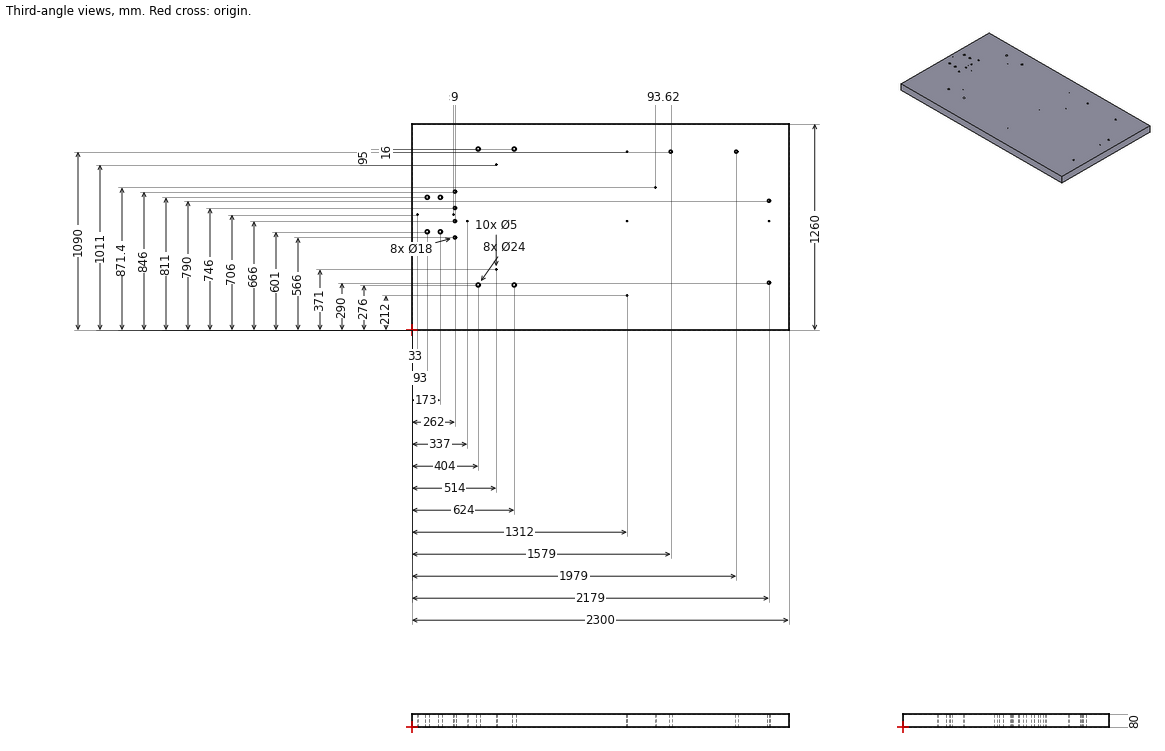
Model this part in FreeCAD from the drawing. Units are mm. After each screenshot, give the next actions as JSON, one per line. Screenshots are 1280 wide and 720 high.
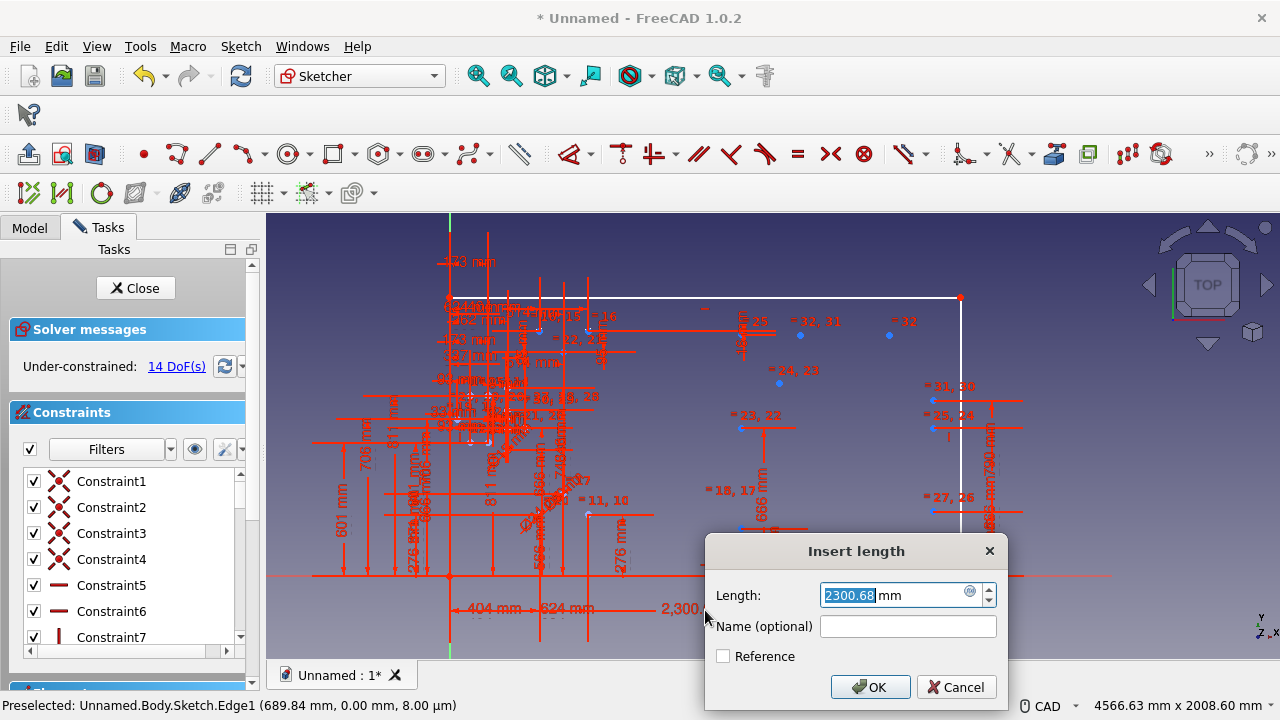
{"action": "type", "text": "2300"}
{"action": "key", "text": "Return"}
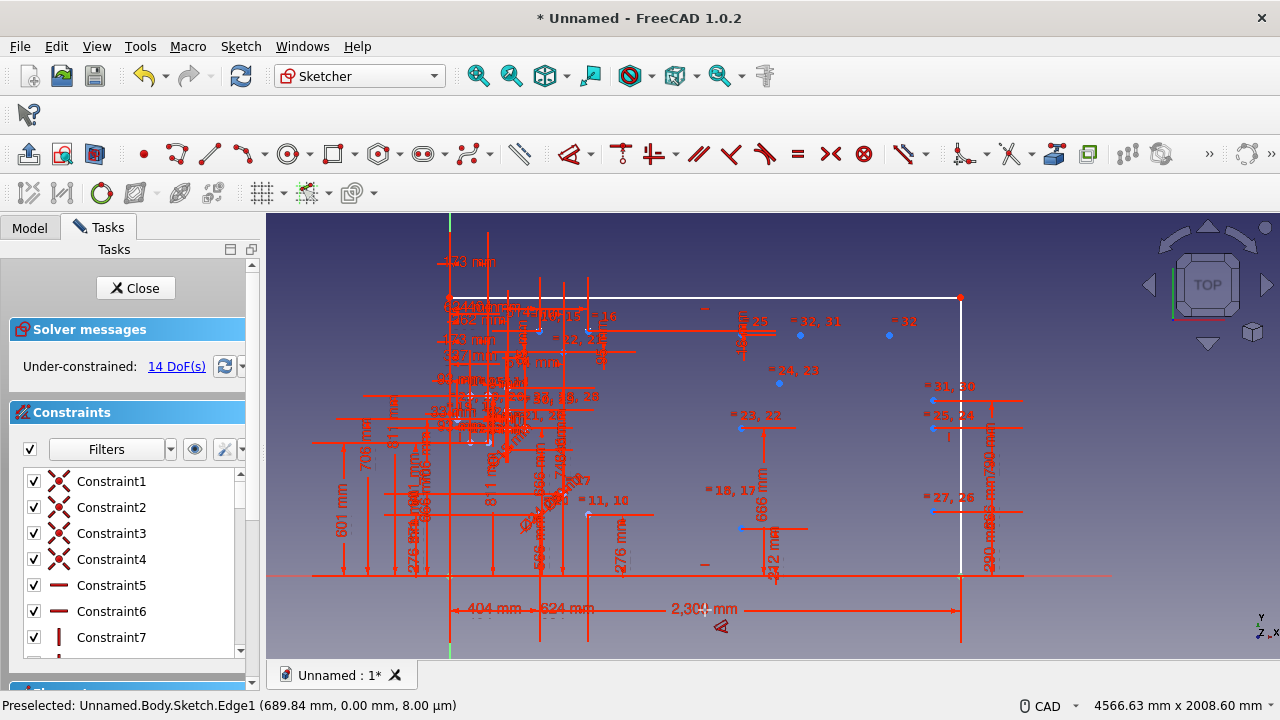
{"action": "left_click", "coordinate": [961, 493]}
{"action": "left_click", "coordinate": [995, 373]}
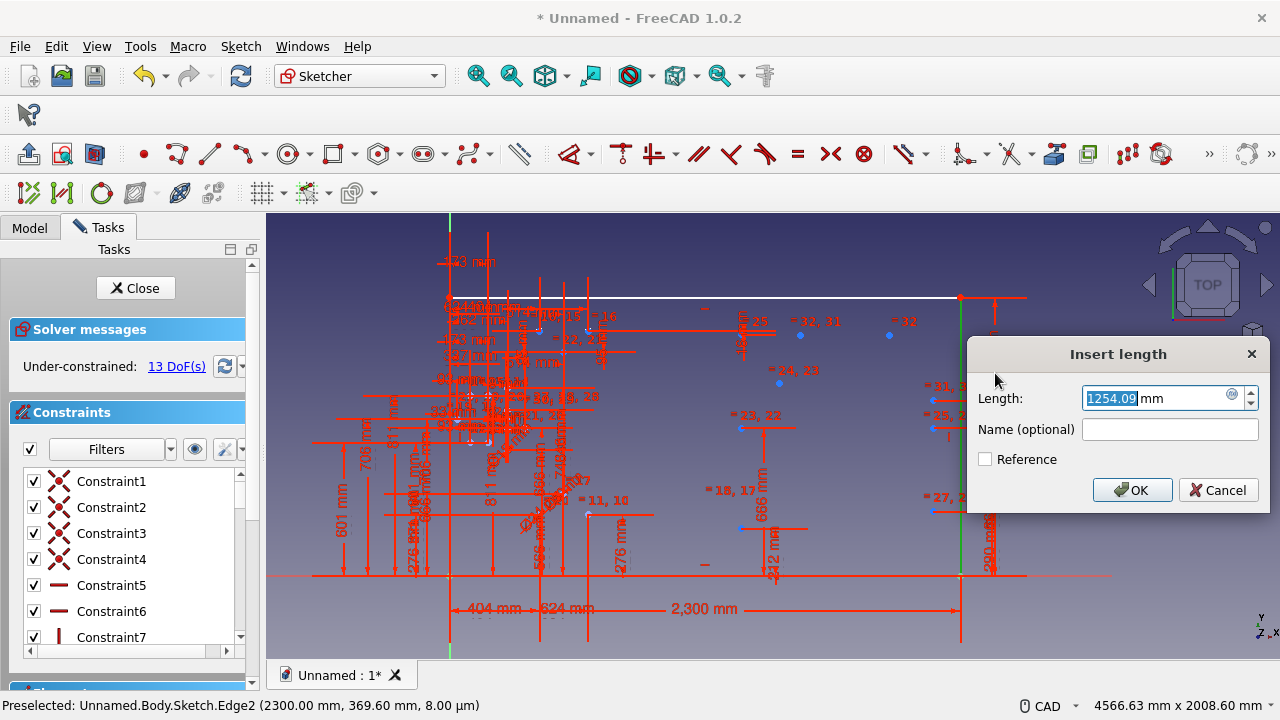
{"action": "type", "text": "1260"}
{"action": "key", "text": "Return"}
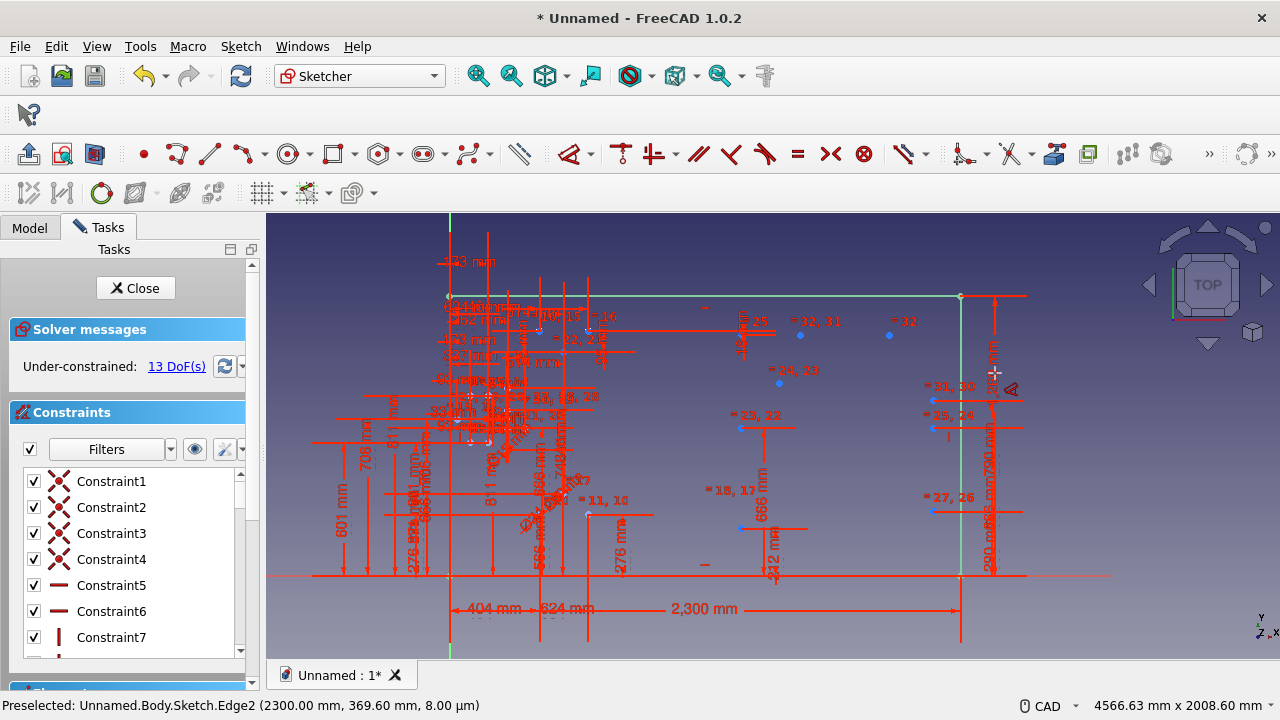
{"action": "left_click", "coordinate": [741, 529]}
{"action": "left_click", "coordinate": [663, 495]}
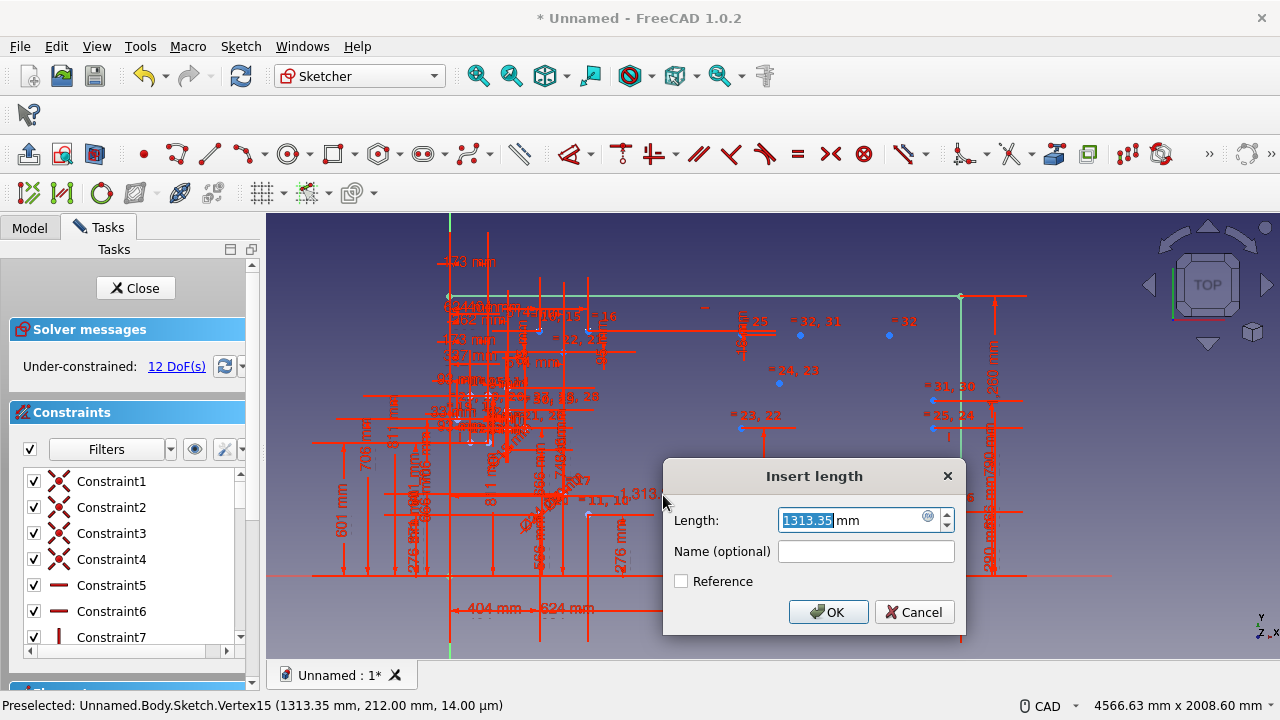
{"action": "type", "text": "1312"}
{"action": "key", "text": "Return"}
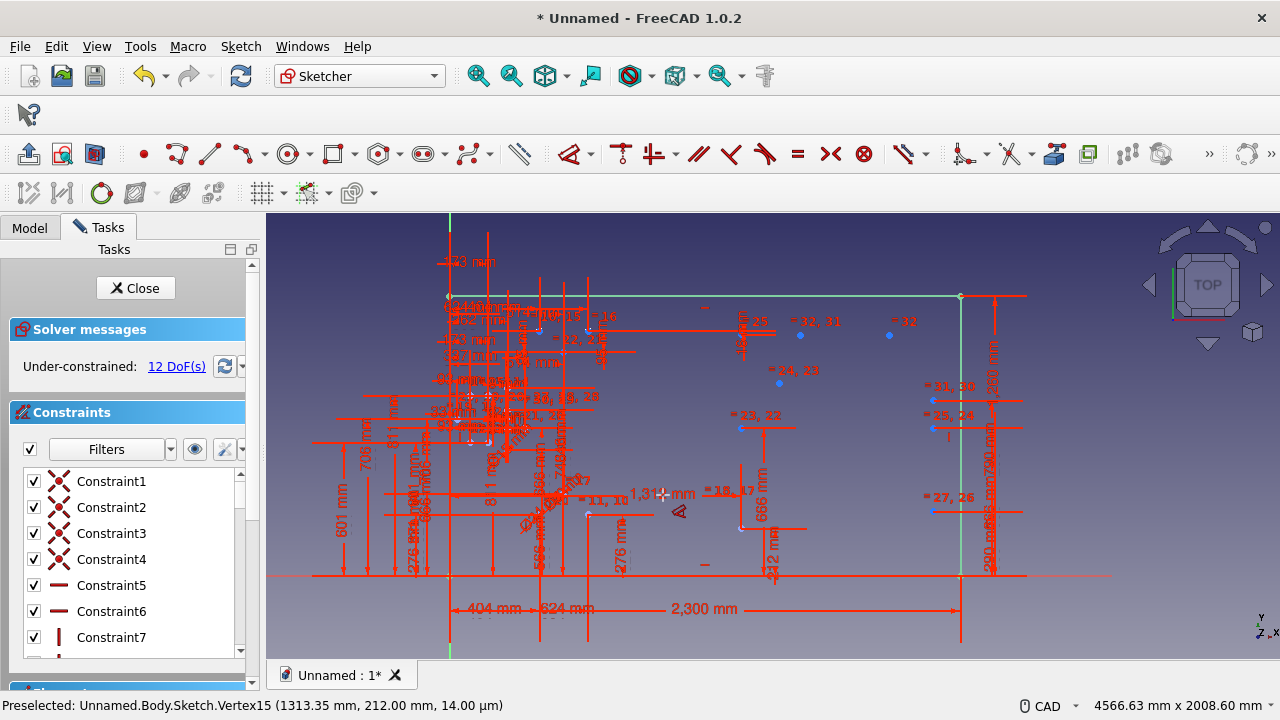
{"action": "left_click", "coordinate": [933, 512]}
{"action": "left_click", "coordinate": [803, 610]}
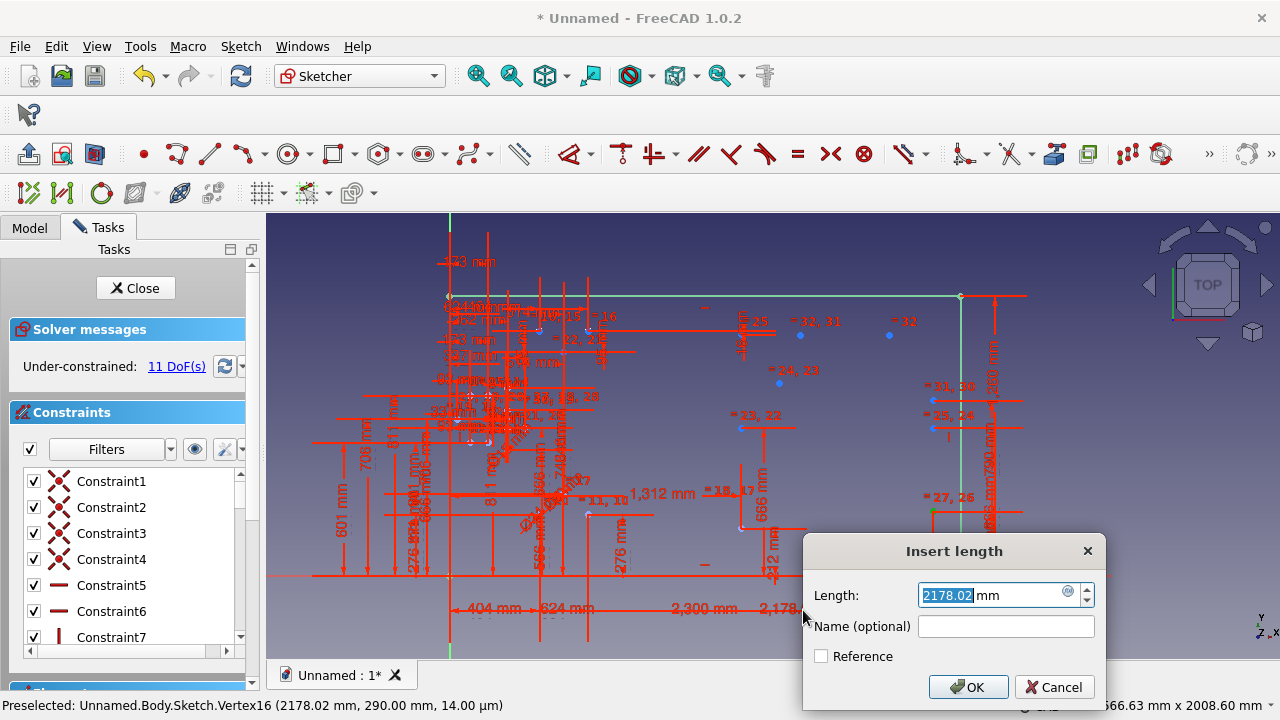
{"action": "type", "text": "2179"}
{"action": "key", "text": "Return"}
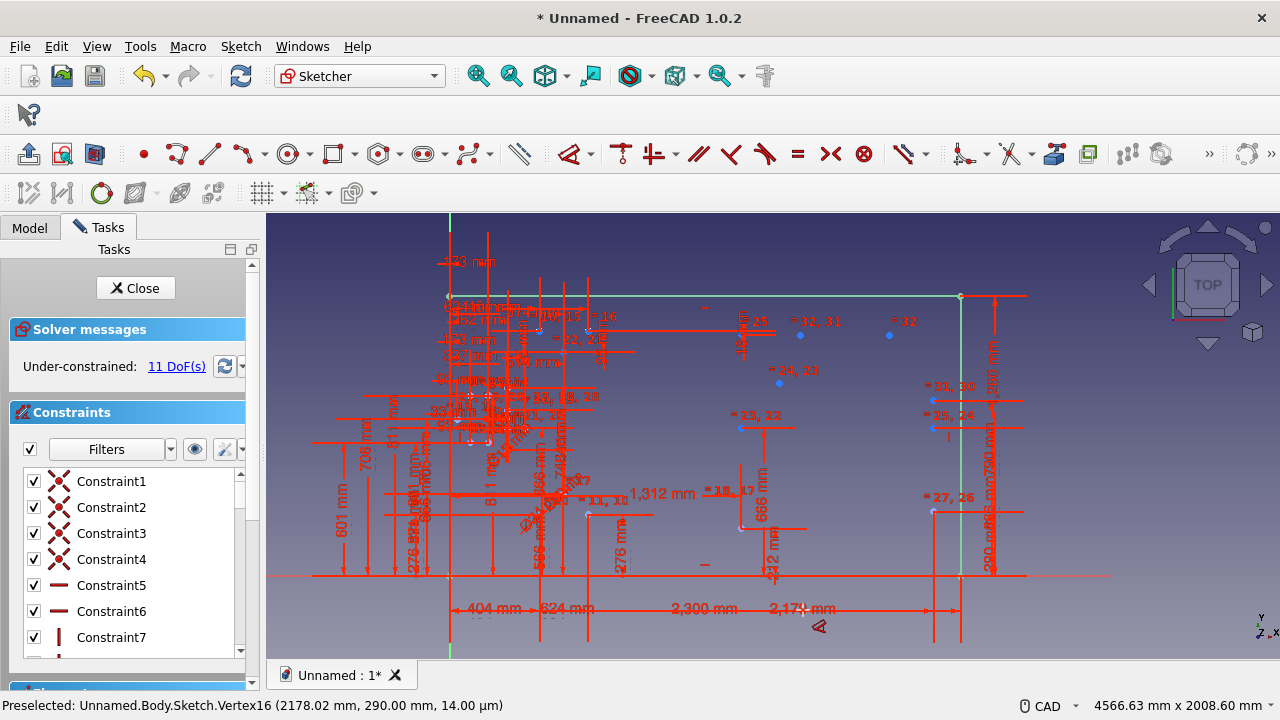
{"action": "left_click", "coordinate": [564, 352]}
{"action": "left_click", "coordinate": [598, 413]}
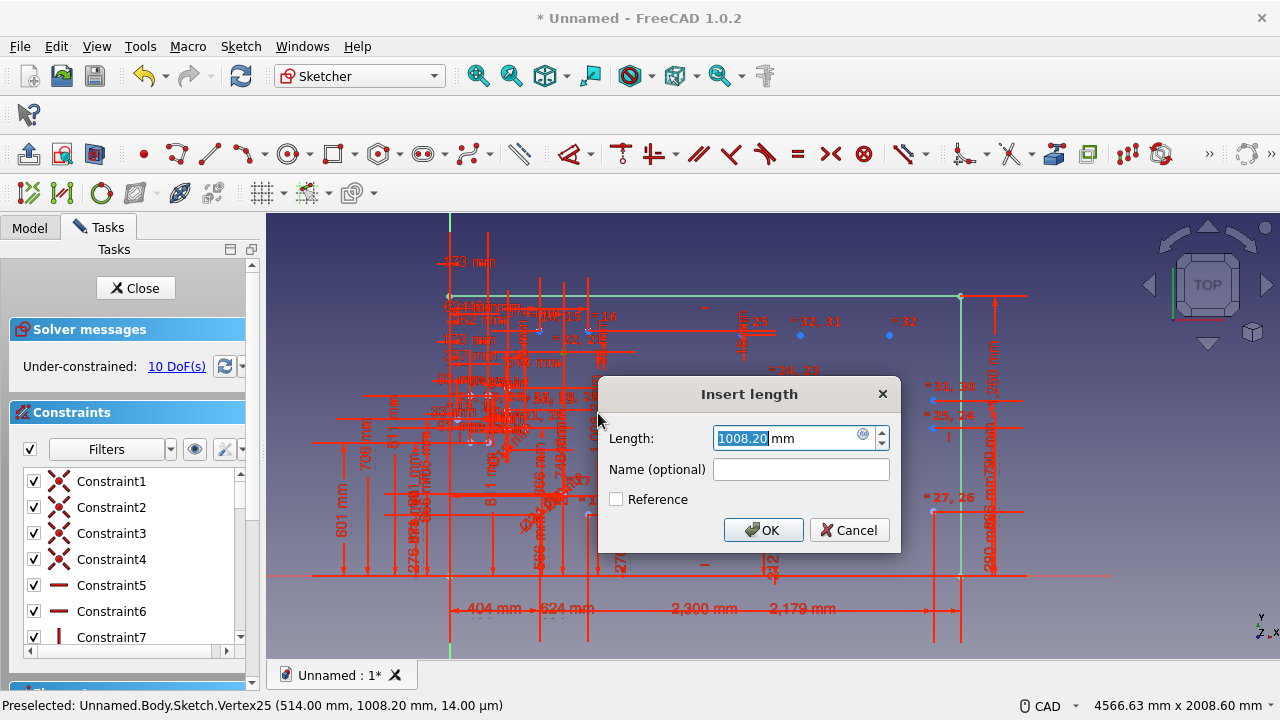
{"action": "type", "text": "1011"}
{"action": "key", "text": "Return"}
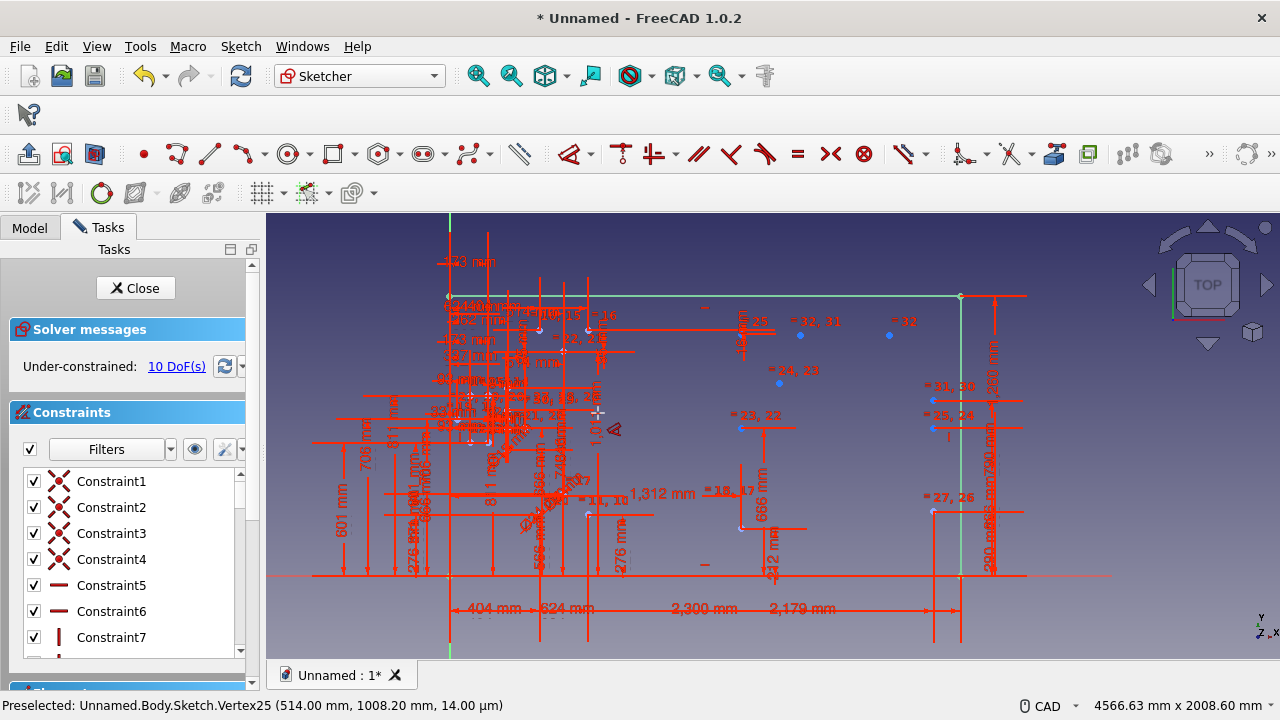
{"action": "left_click", "coordinate": [741, 428]}
{"action": "left_click", "coordinate": [697, 394]}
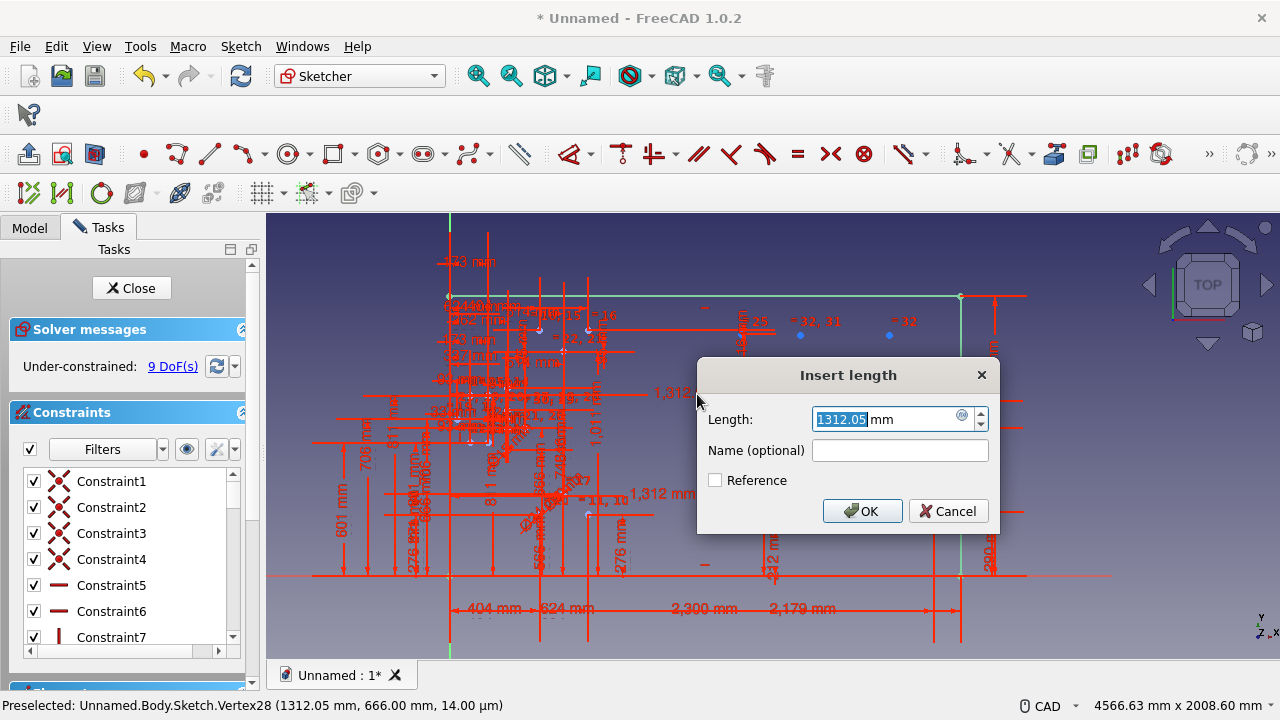
{"action": "type", "text": "1312"}
{"action": "key", "text": "Return"}